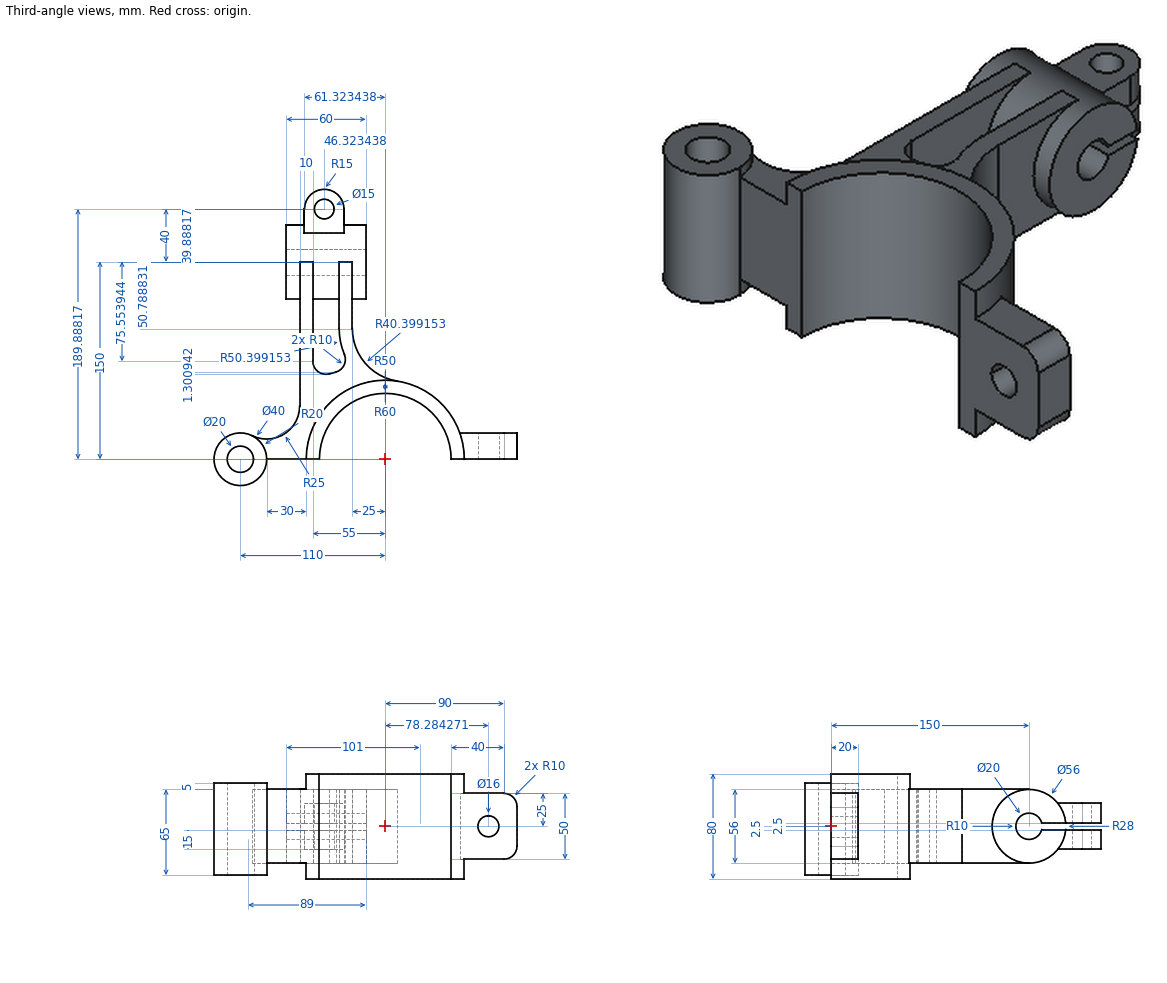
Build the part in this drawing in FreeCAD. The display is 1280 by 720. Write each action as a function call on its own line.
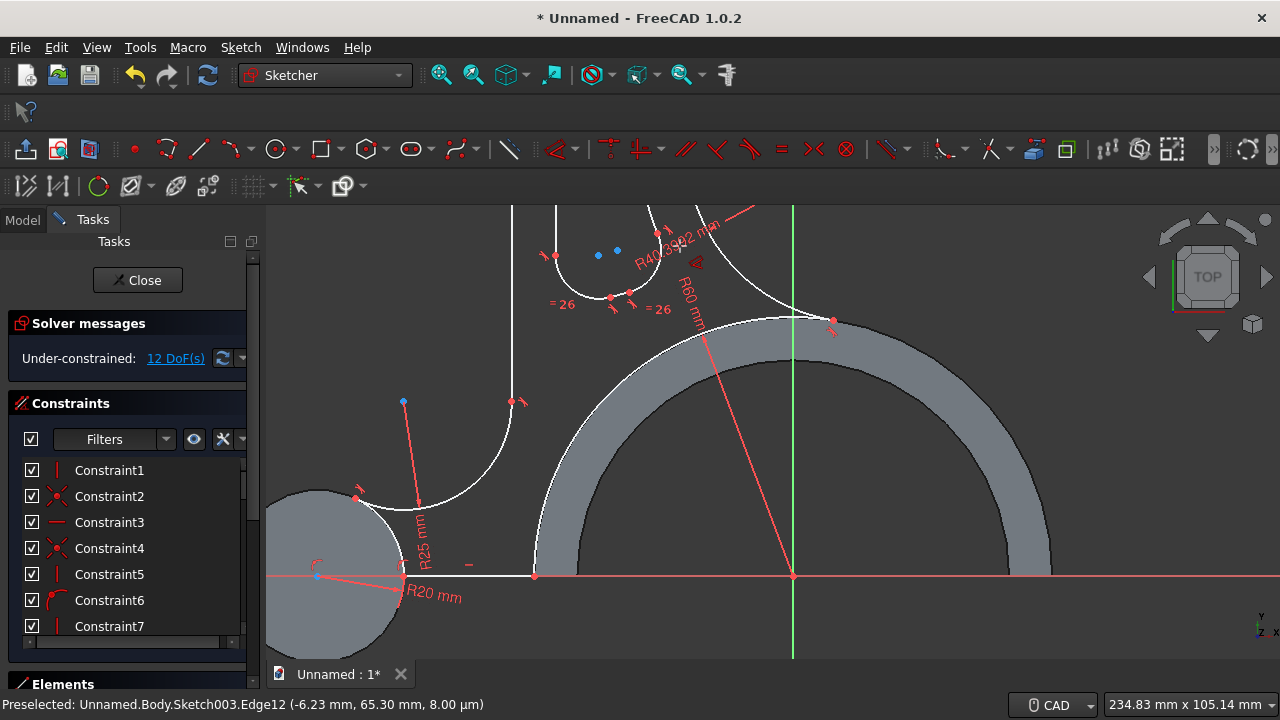
scroll(794, 579, down, 4)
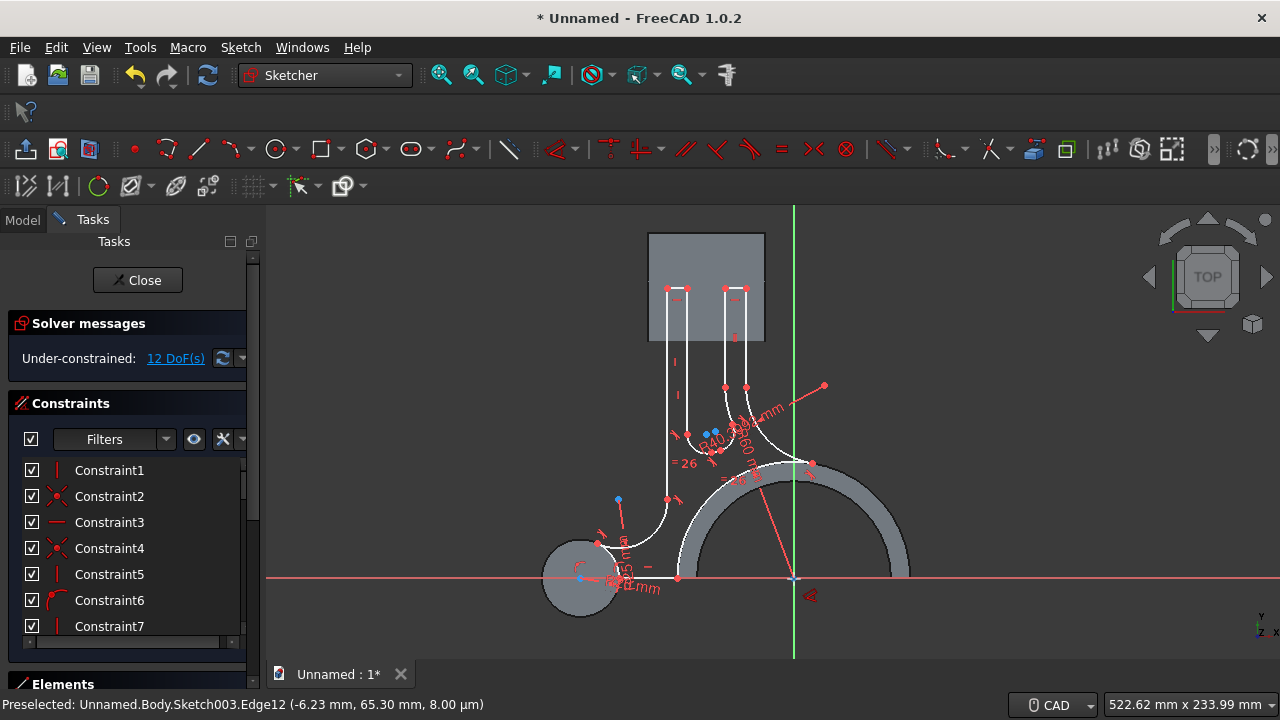
click(726, 398)
click(702, 338)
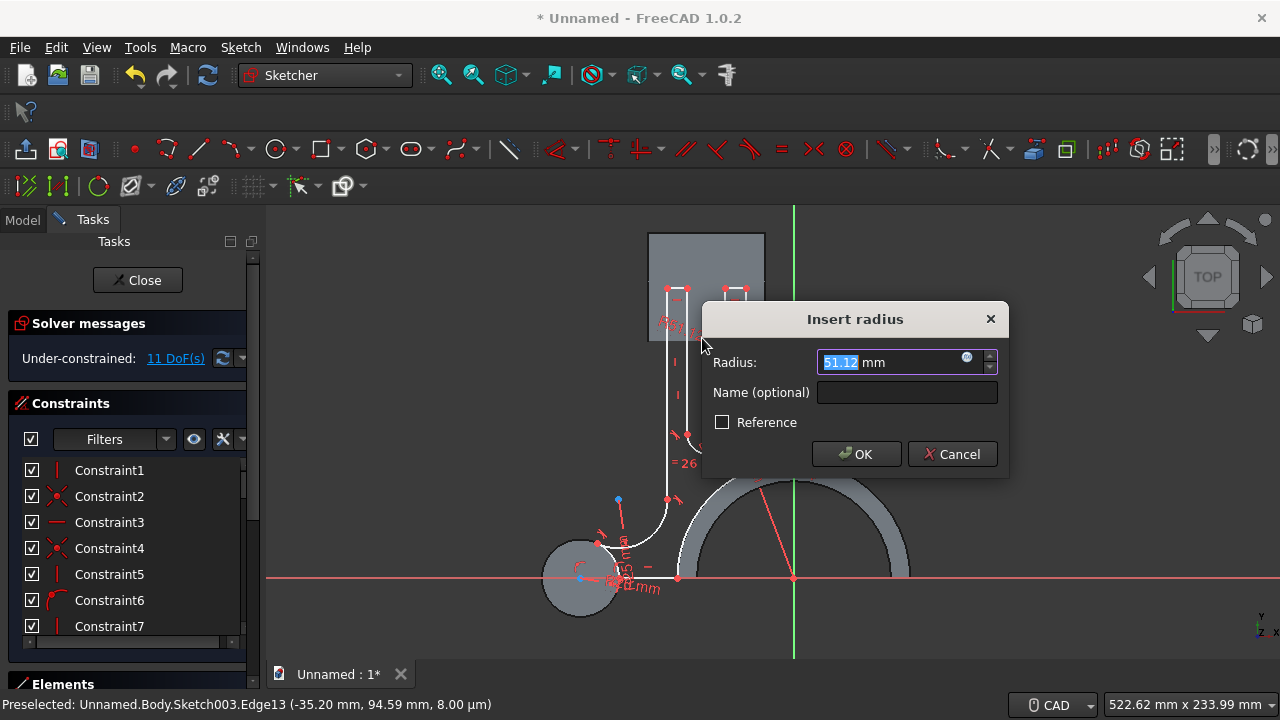
text(50.399153)
key(Return)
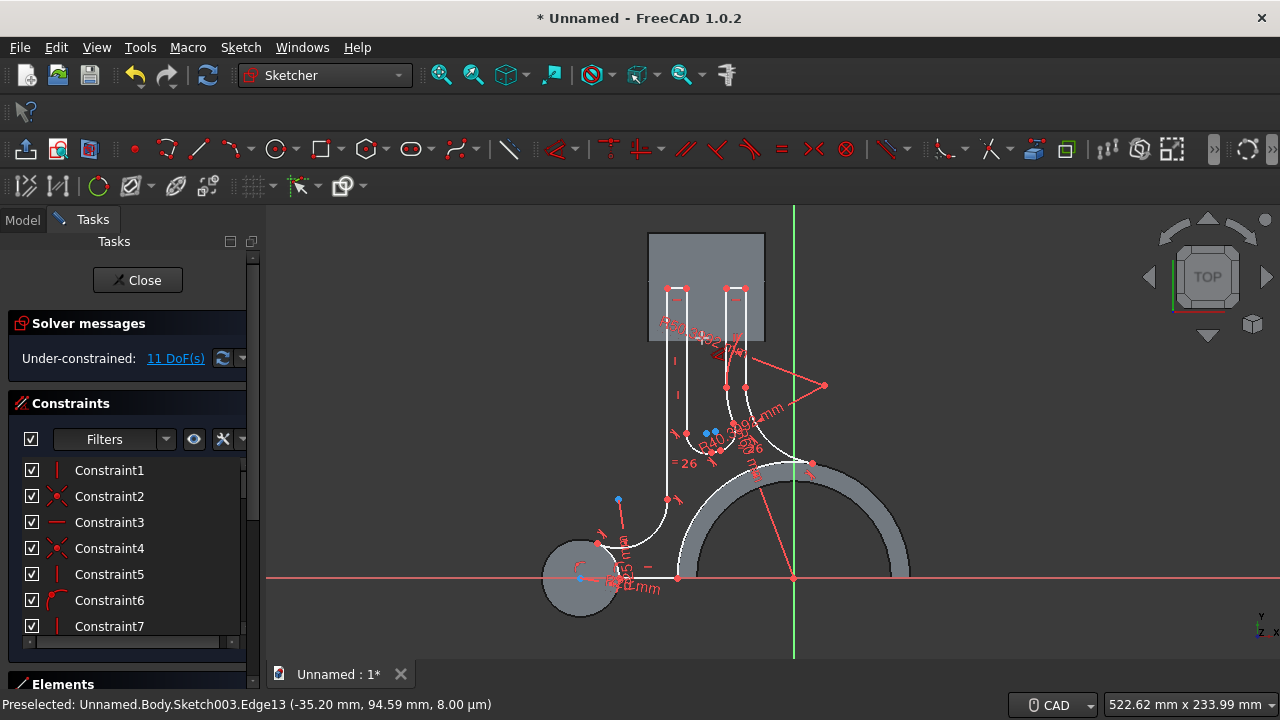
scroll(729, 446, up, 4)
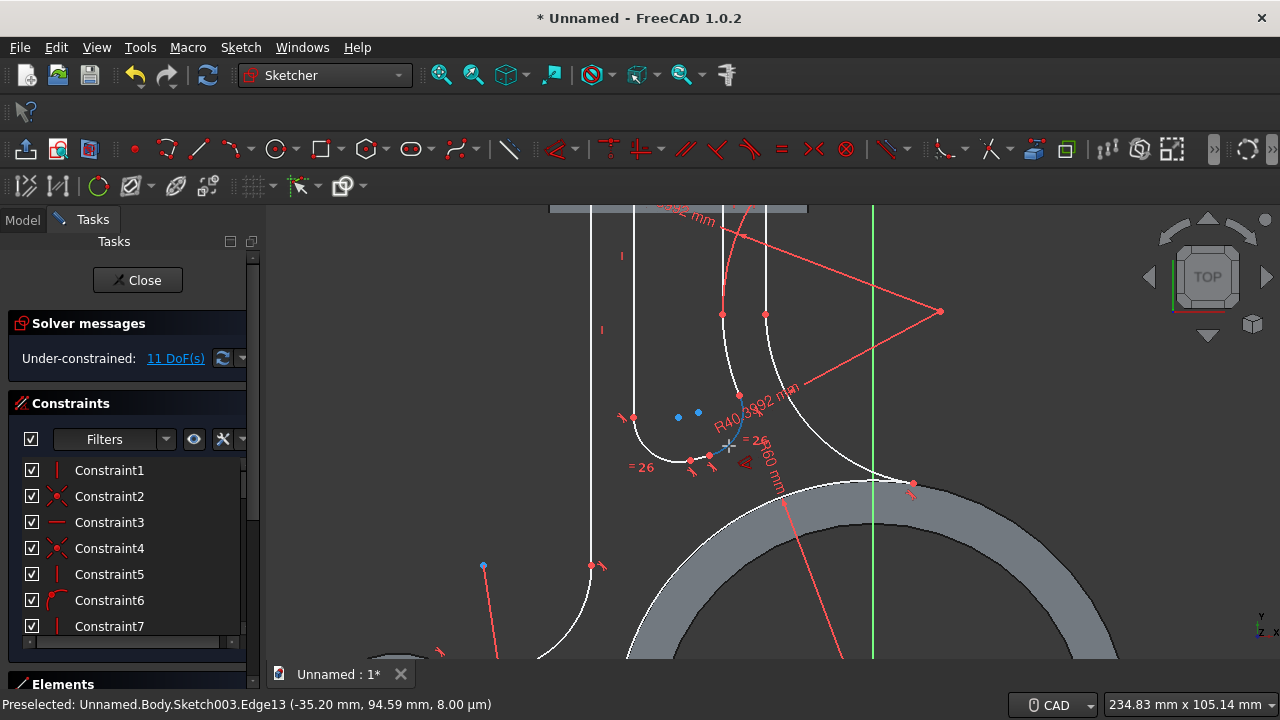
click(729, 444)
click(771, 435)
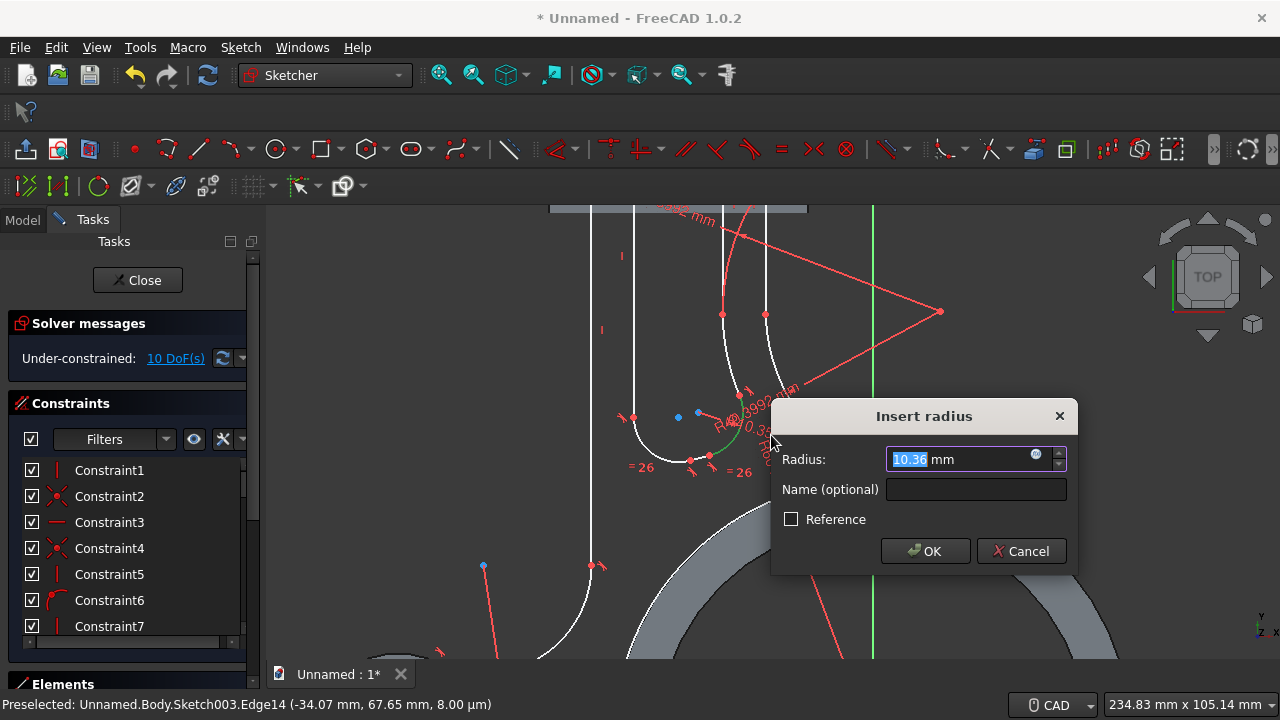
text(10)
key(Return)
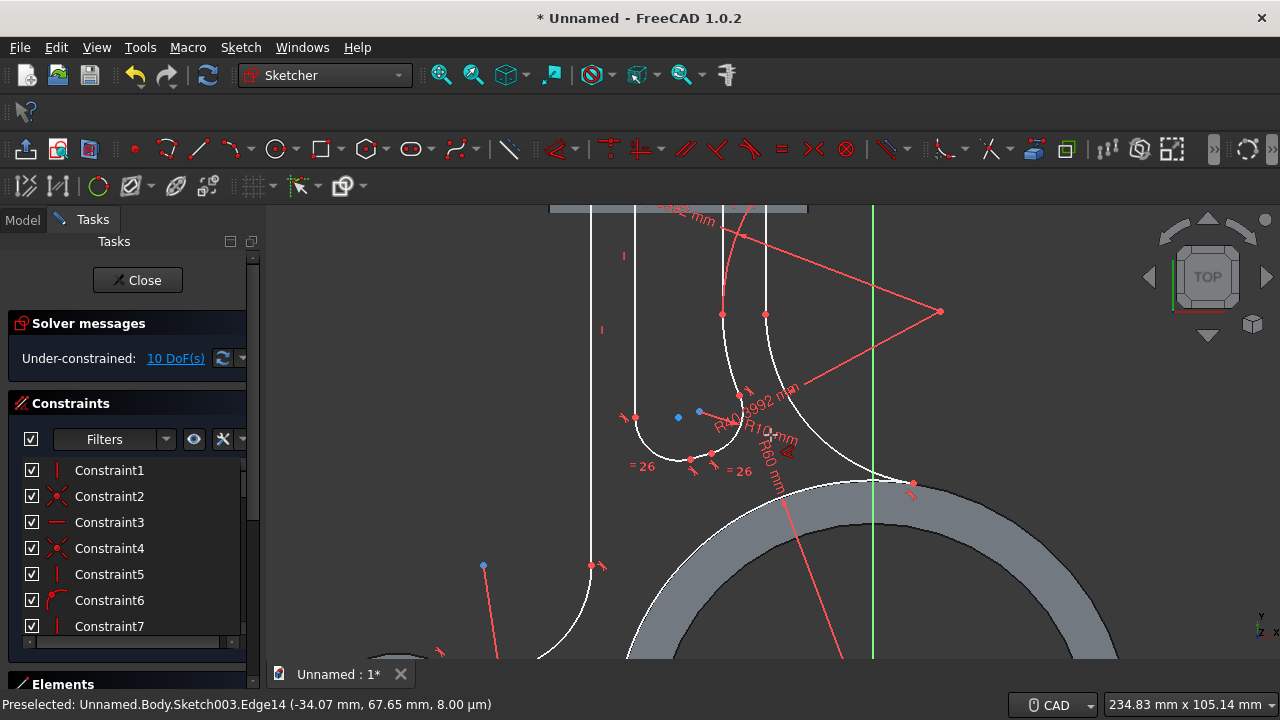
scroll(729, 445, down, 4)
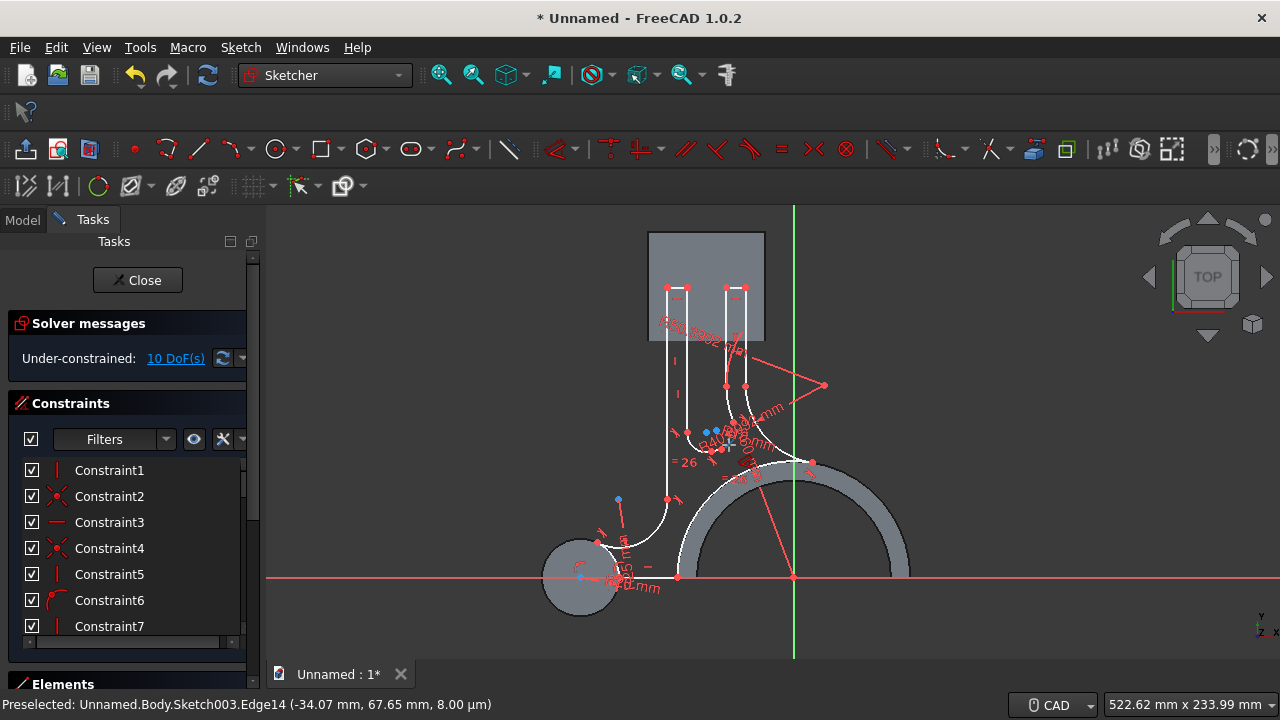
scroll(681, 288, up, 5)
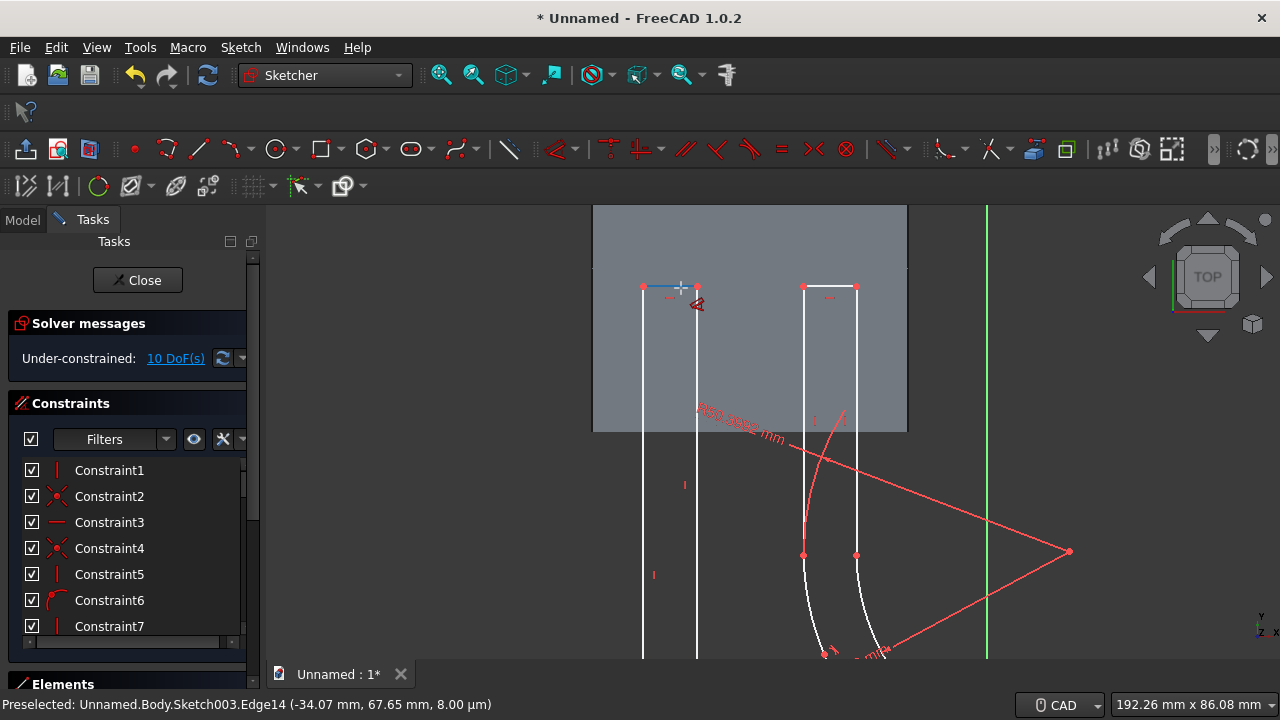
click(681, 286)
click(670, 252)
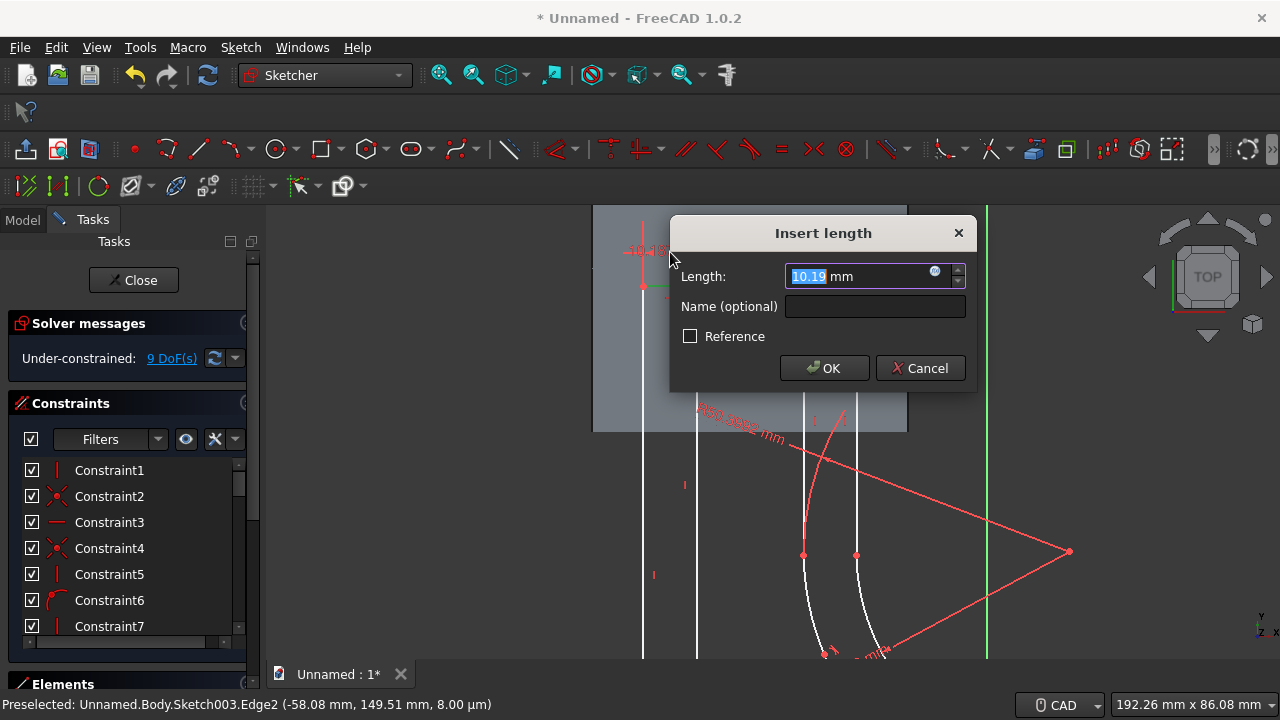
text(10)
key(Return)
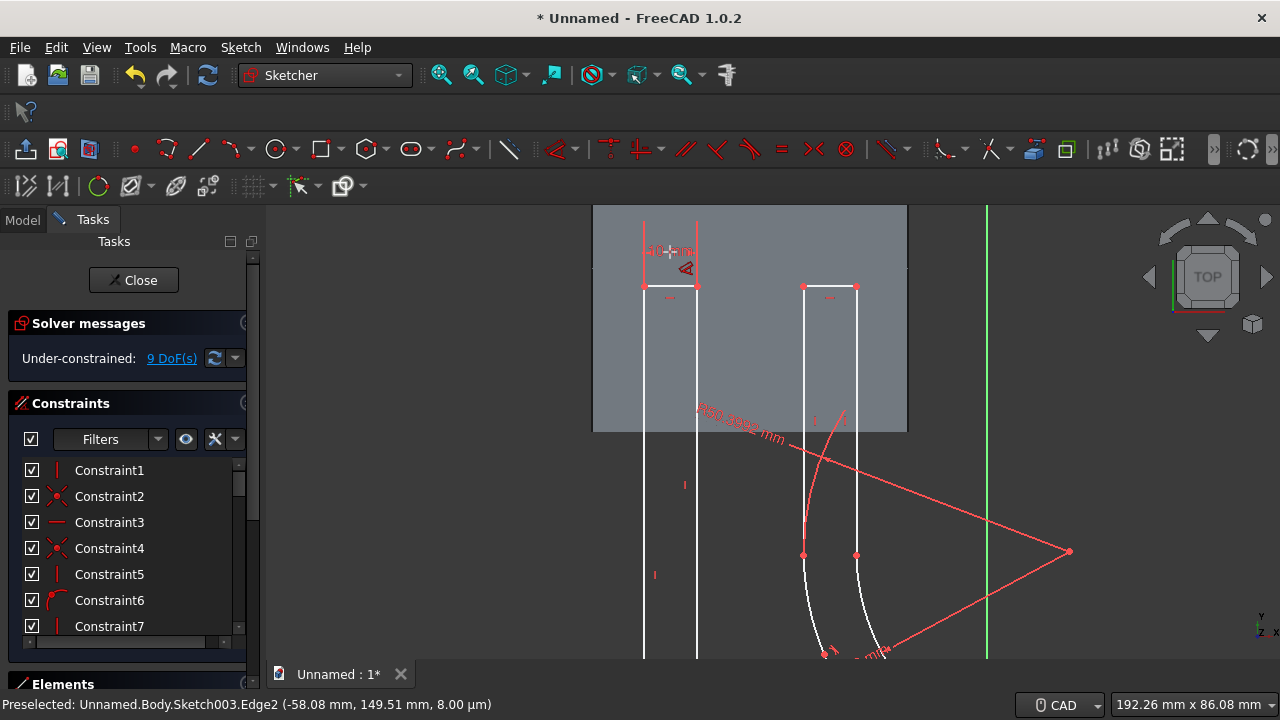
scroll(681, 288, down, 5)